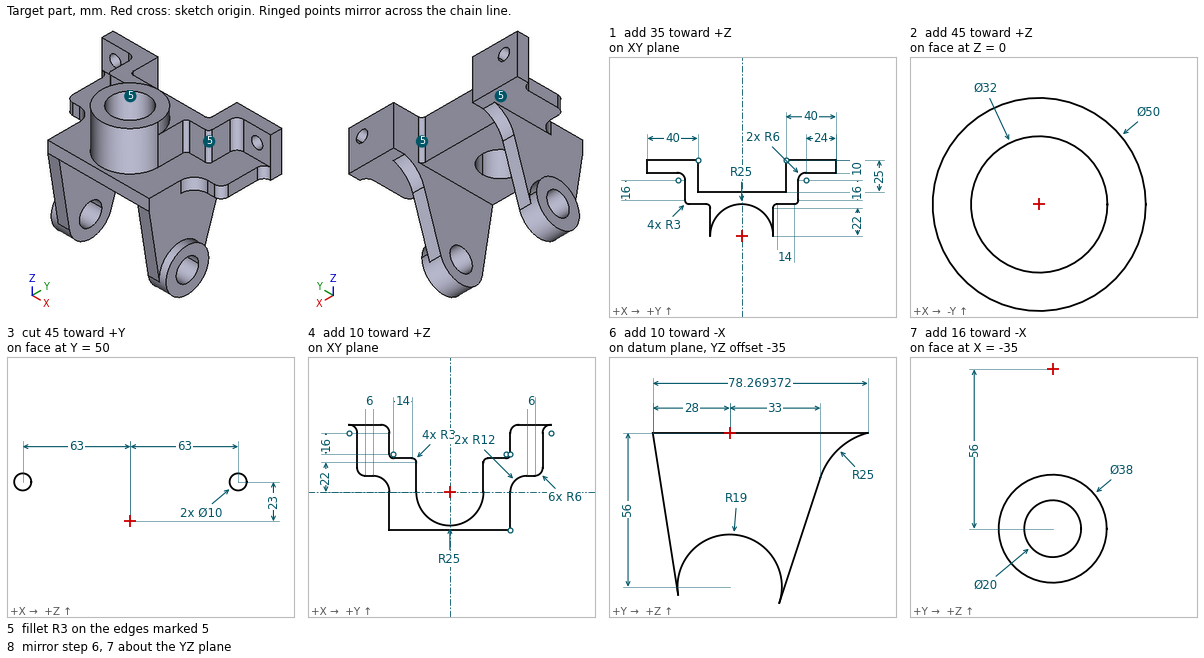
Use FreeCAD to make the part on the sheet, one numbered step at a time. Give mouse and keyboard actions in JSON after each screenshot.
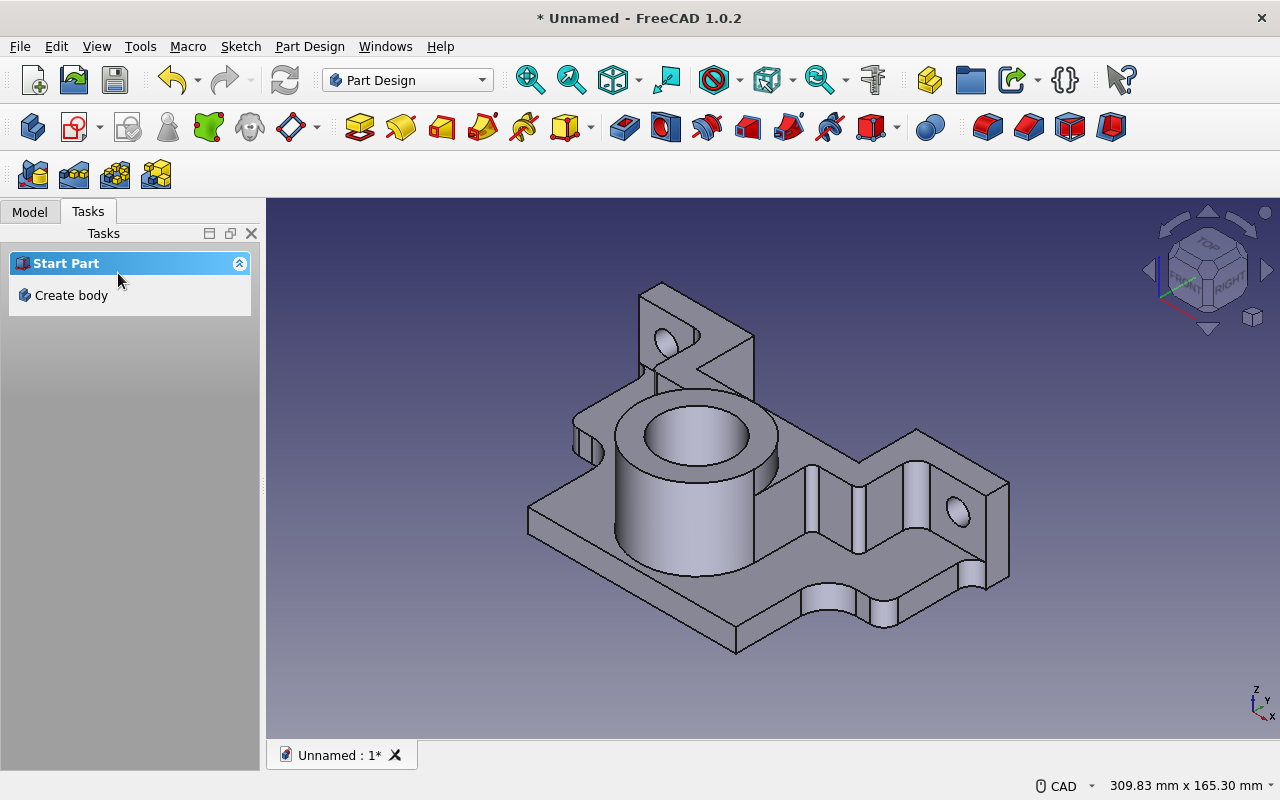
{"action": "key", "text": "2"}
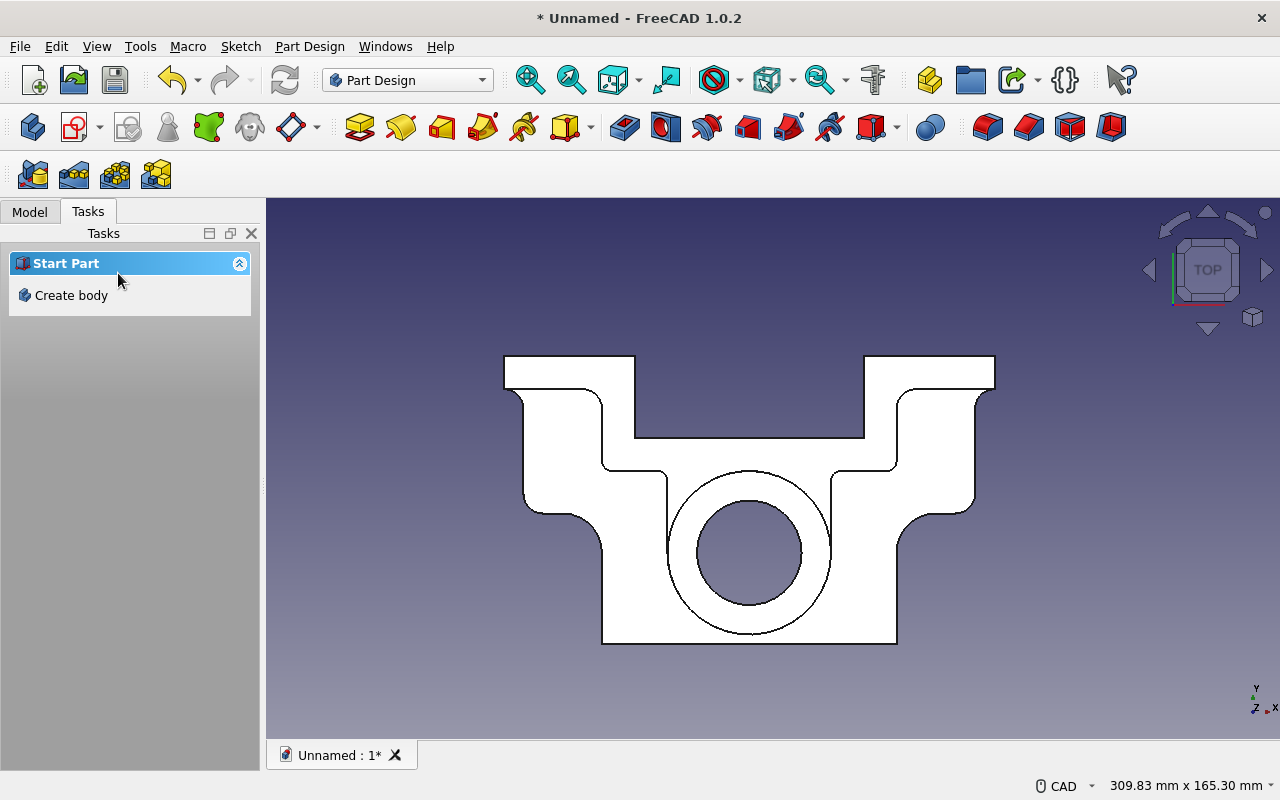
{"action": "key", "text": "0"}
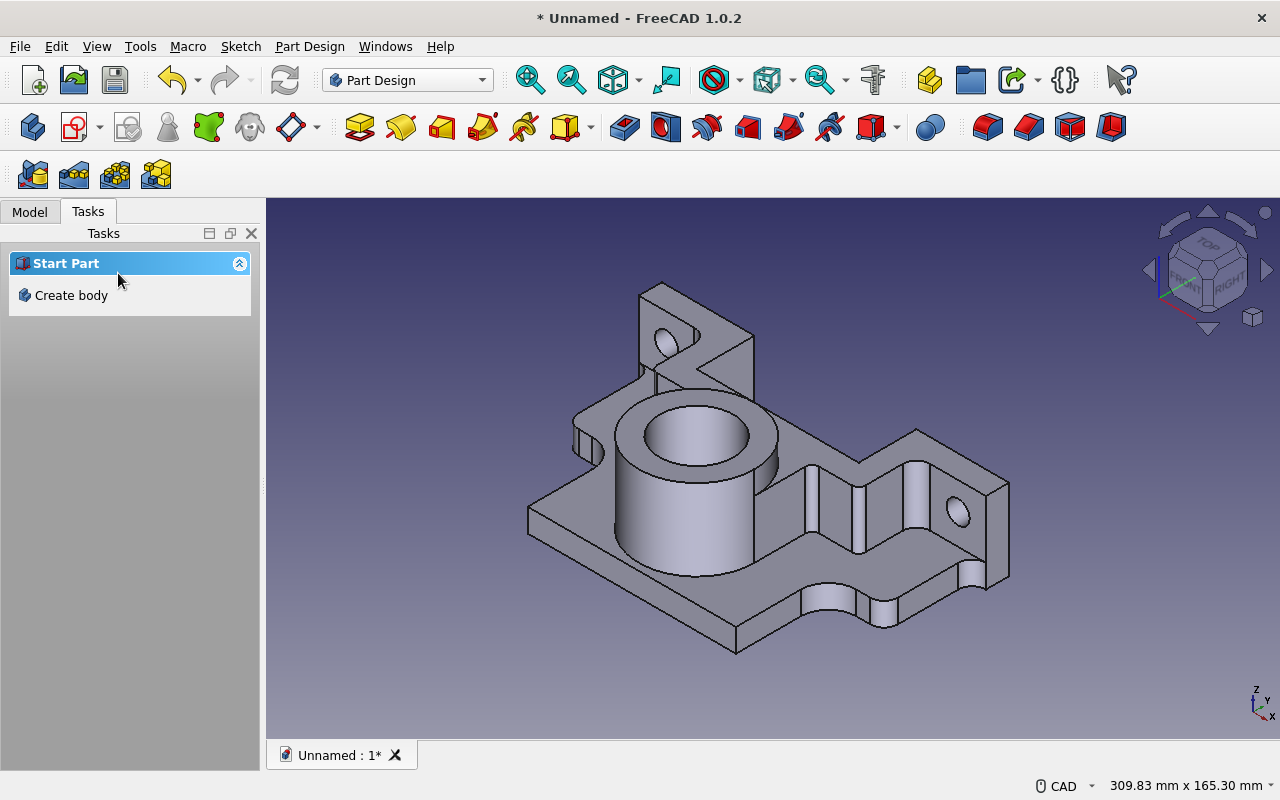
{"action": "key", "text": "1"}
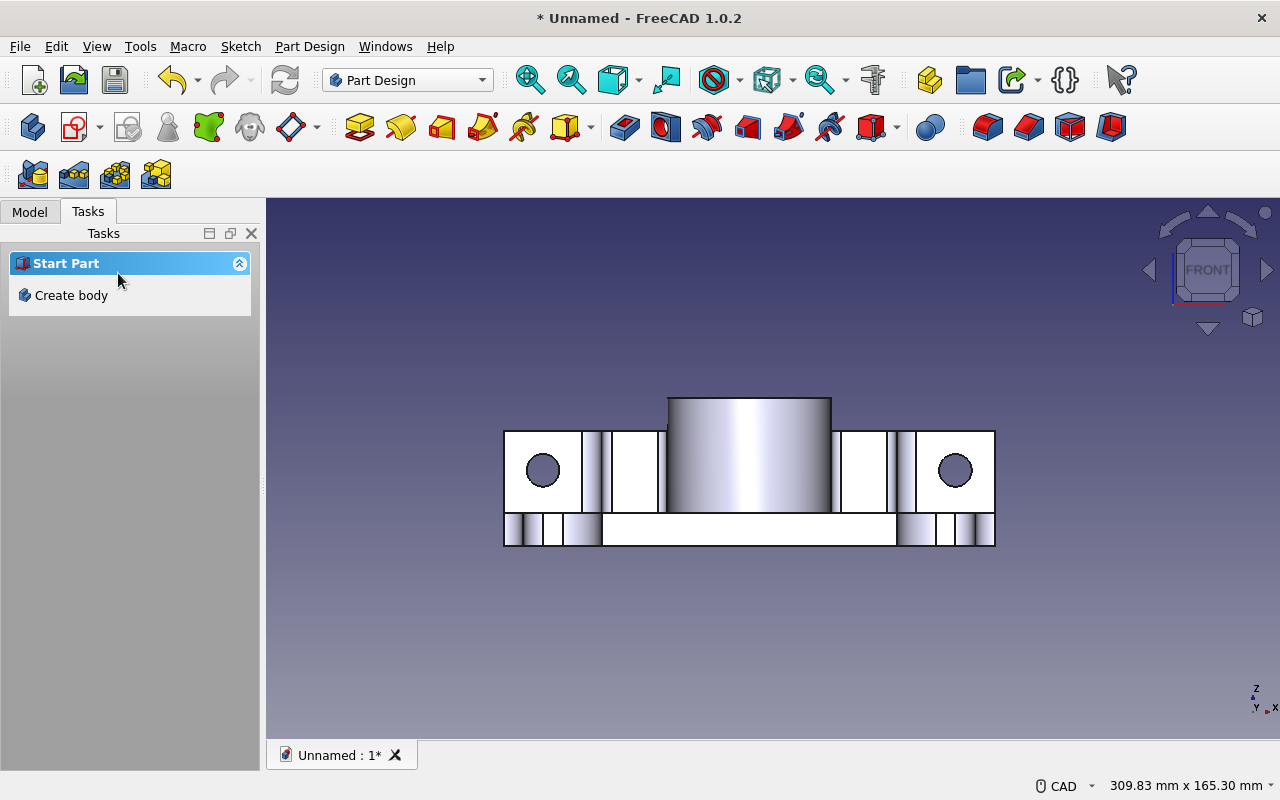
{"action": "key", "text": "3"}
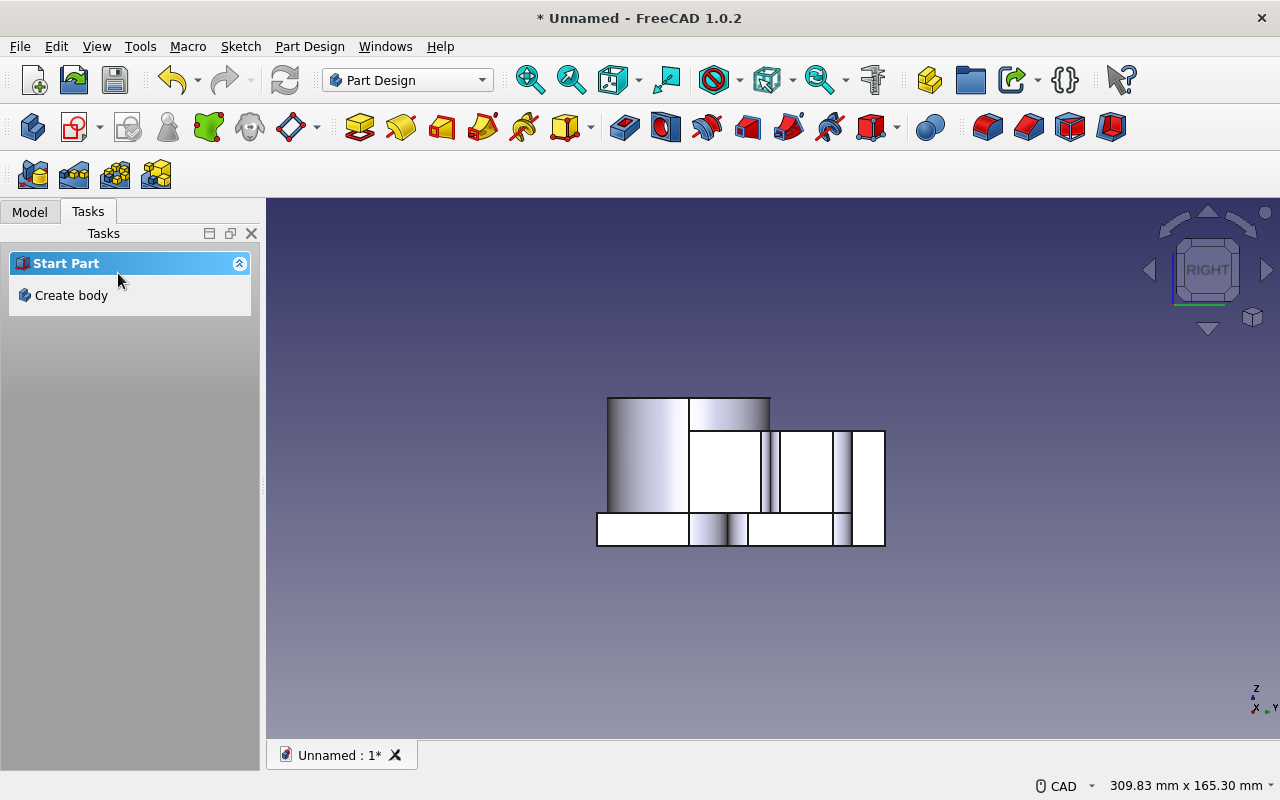
{"action": "left_click", "coordinate": [531, 80]}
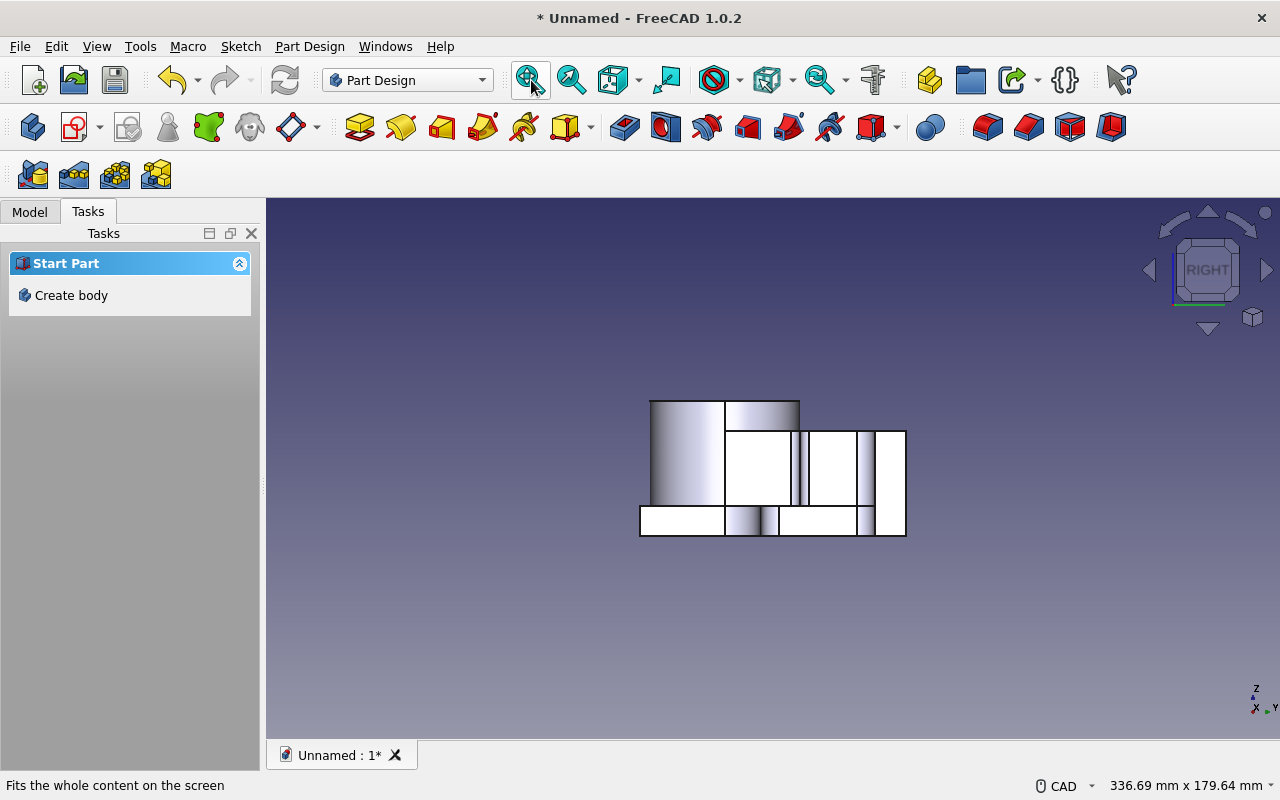
{"action": "key", "text": "5"}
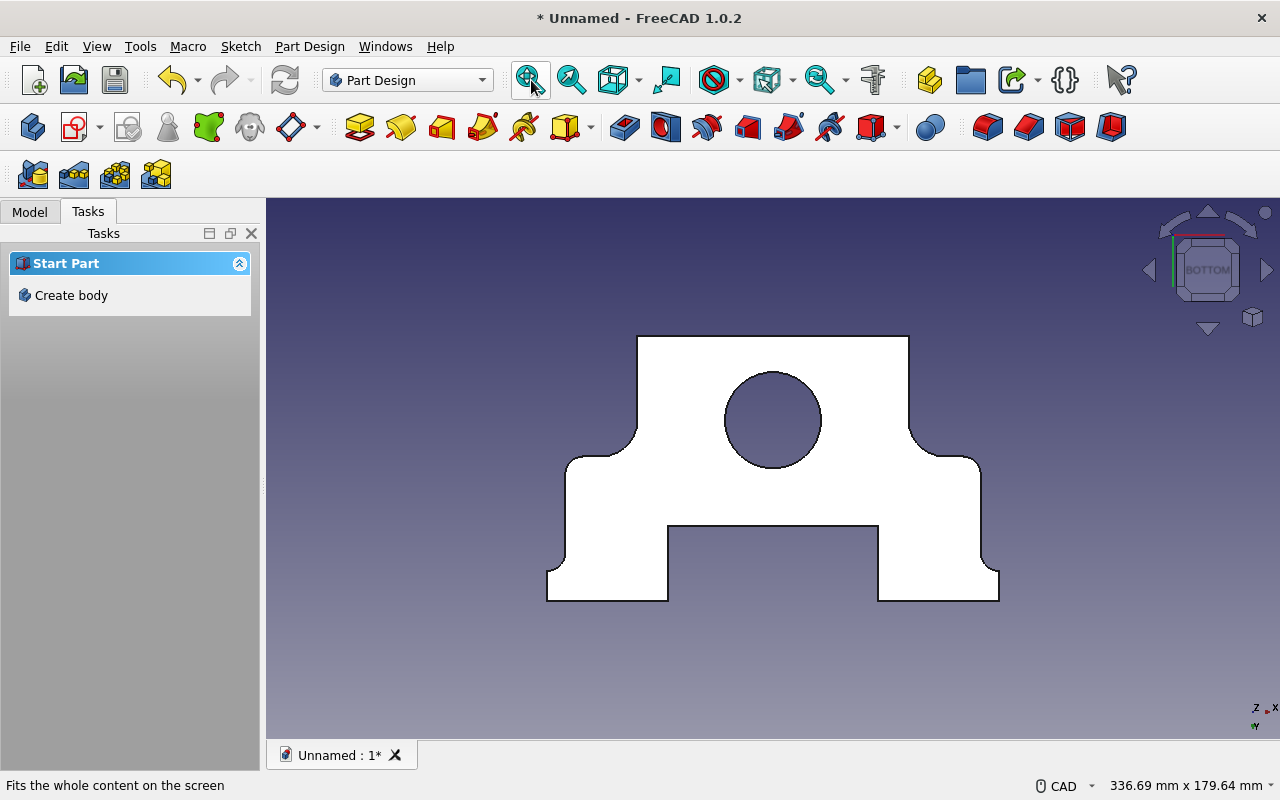
{"action": "key", "text": "4"}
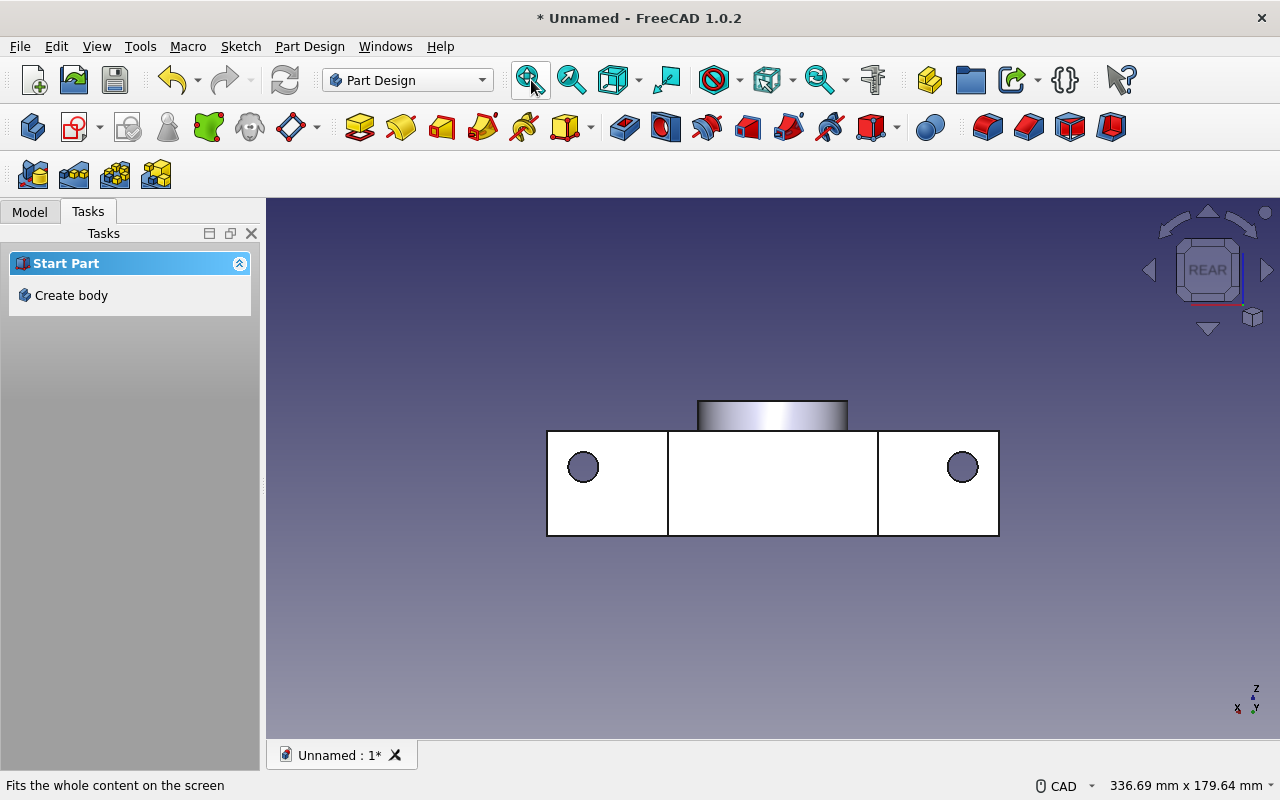
{"action": "left_click", "coordinate": [531, 80]}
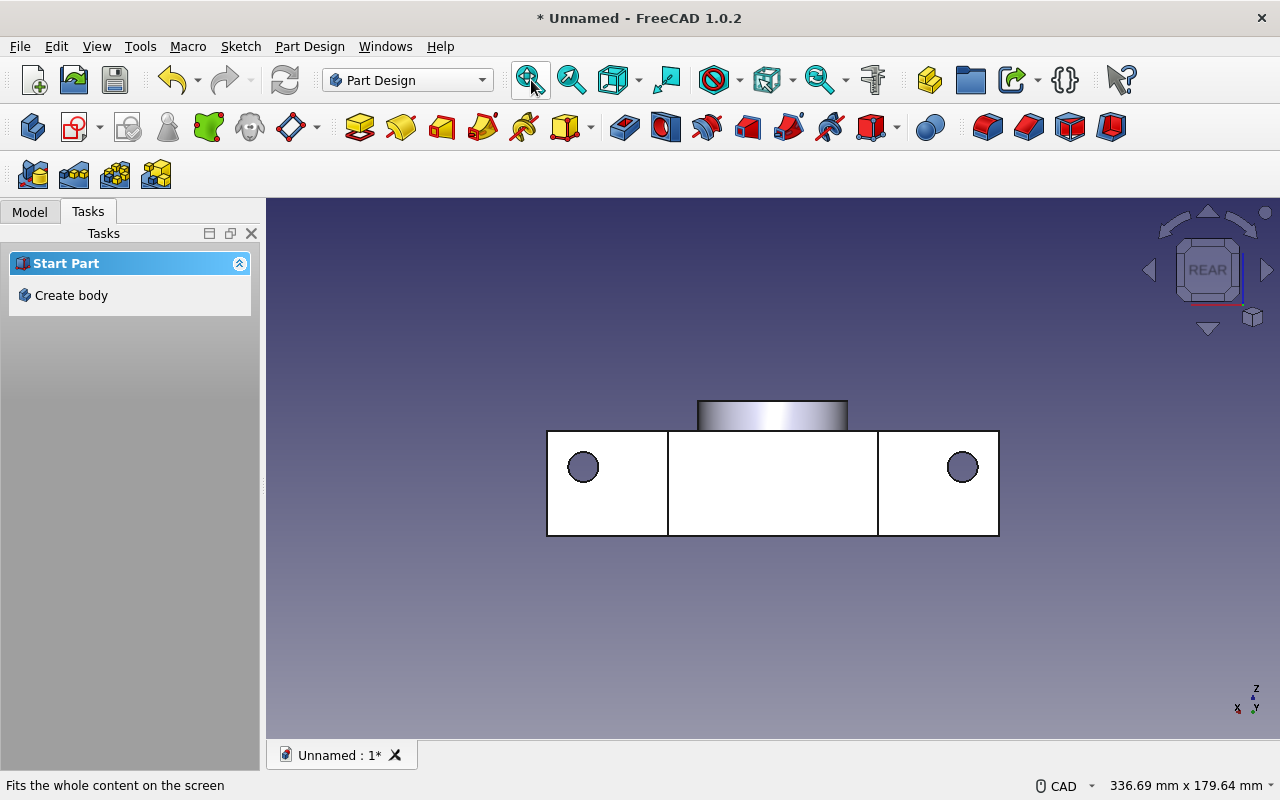
{"action": "key", "text": "6"}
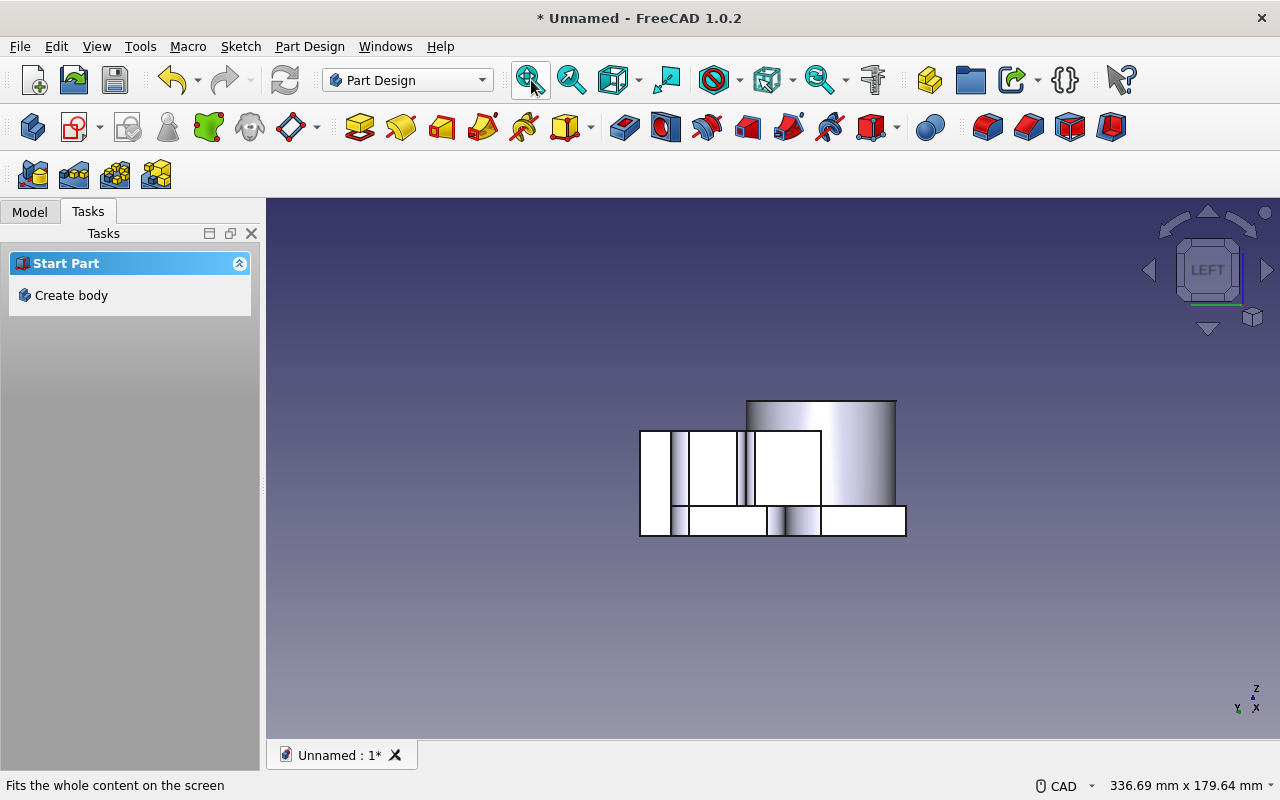
{"action": "left_click", "coordinate": [531, 80]}